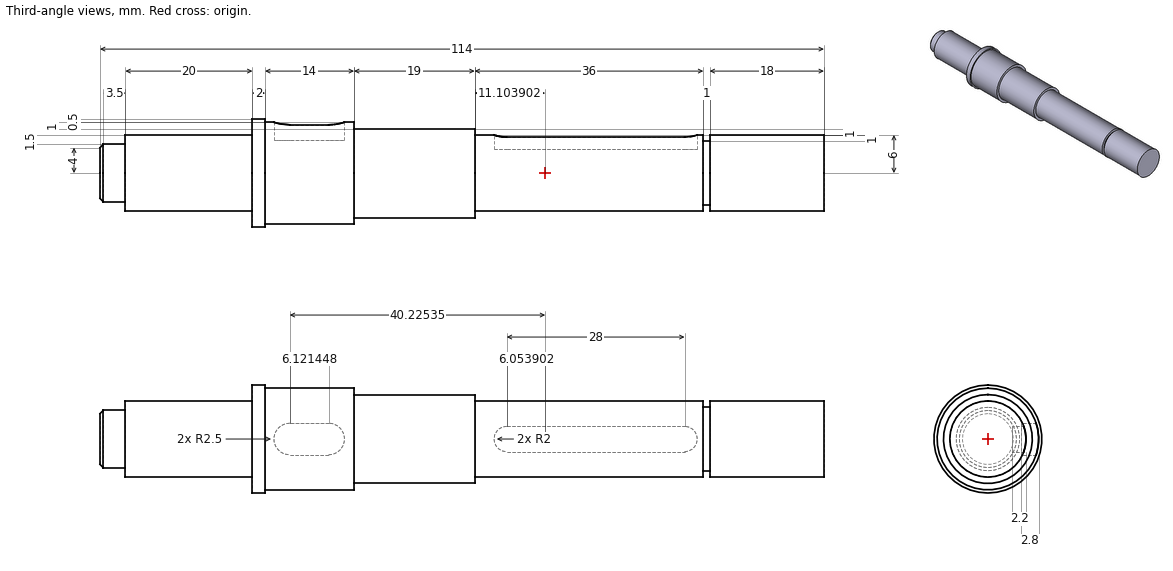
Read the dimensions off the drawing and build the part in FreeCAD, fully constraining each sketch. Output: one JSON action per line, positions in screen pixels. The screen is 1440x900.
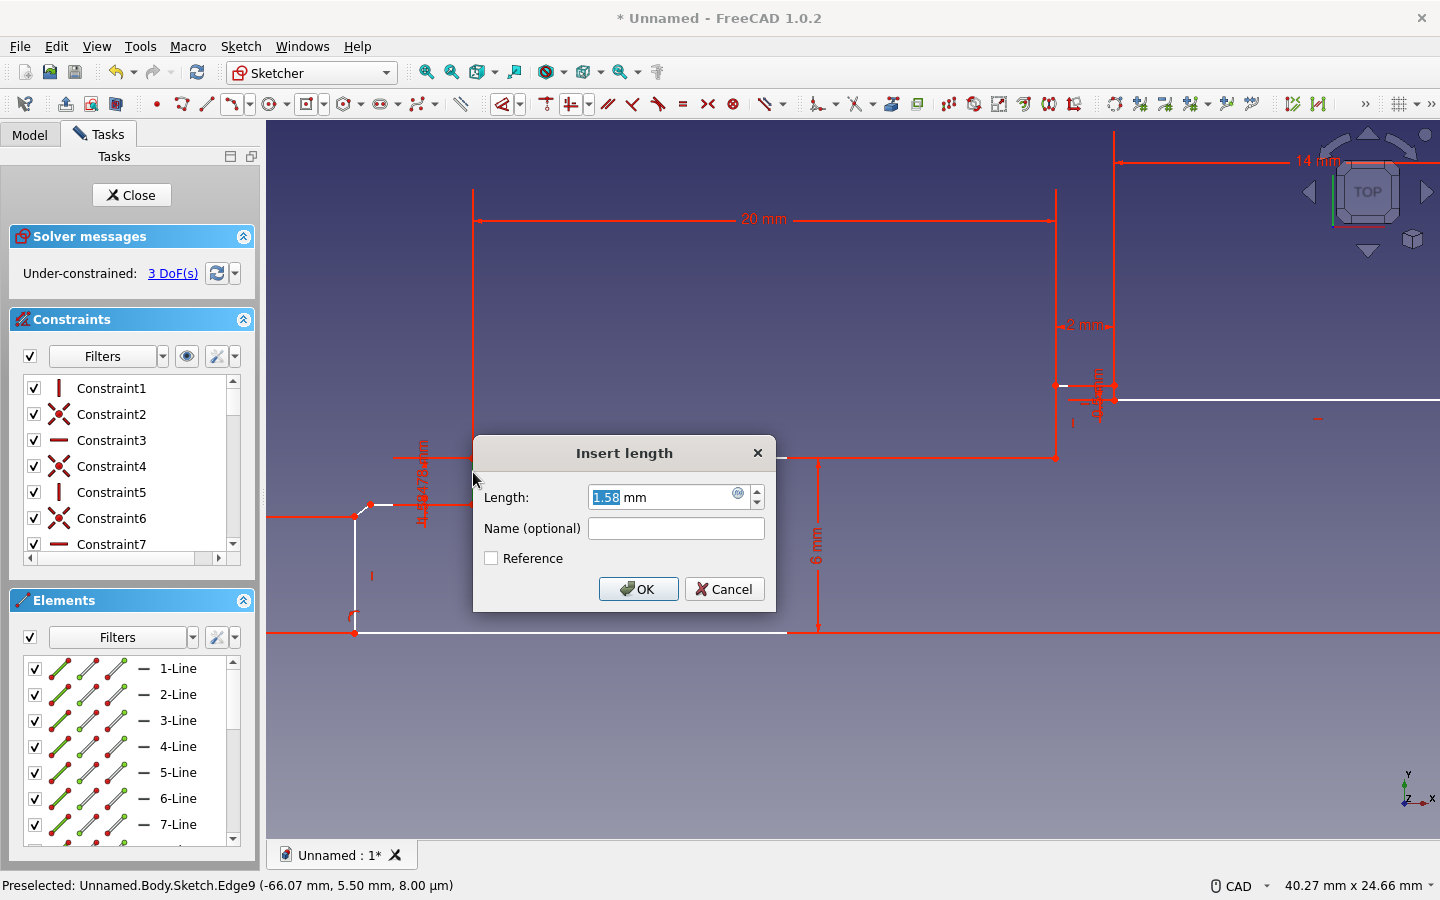
{"action": "type", "text": "1.5"}
{"action": "key", "text": "Return"}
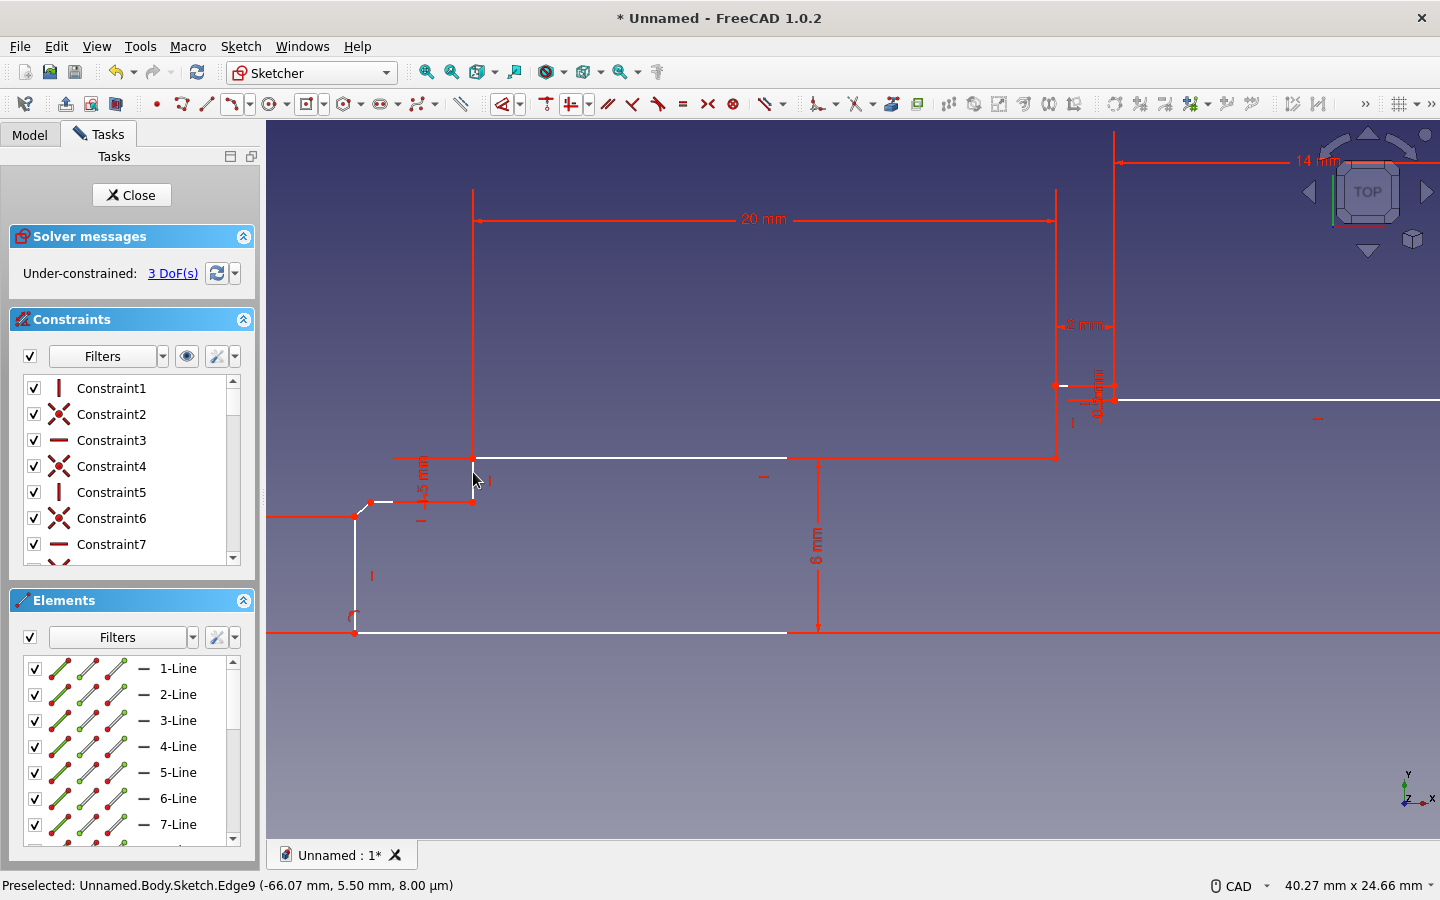
{"action": "left_click", "coordinate": [442, 502]}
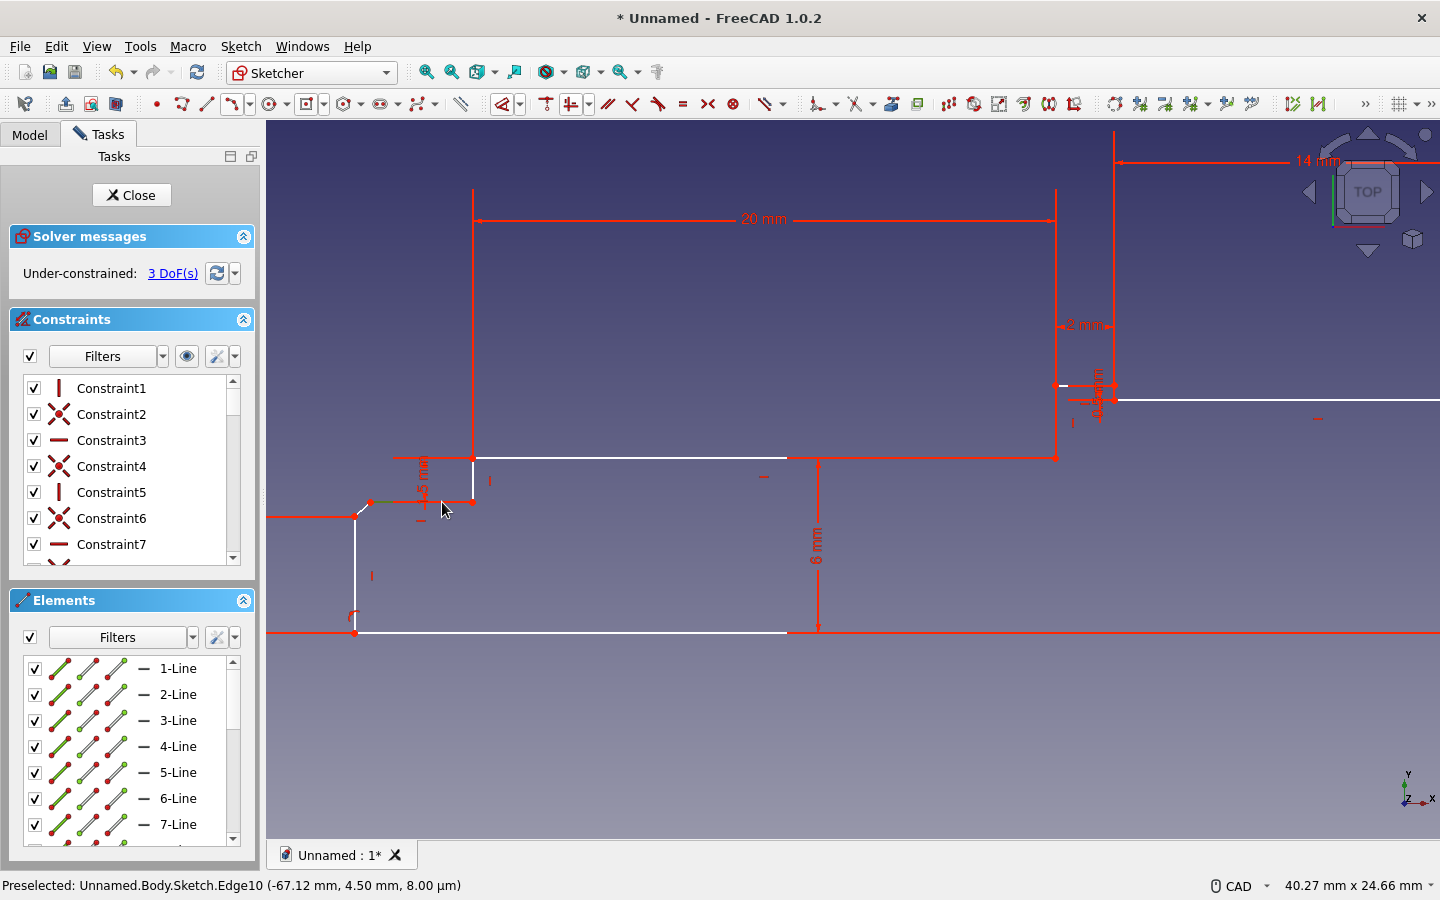
{"action": "key", "text": "l"}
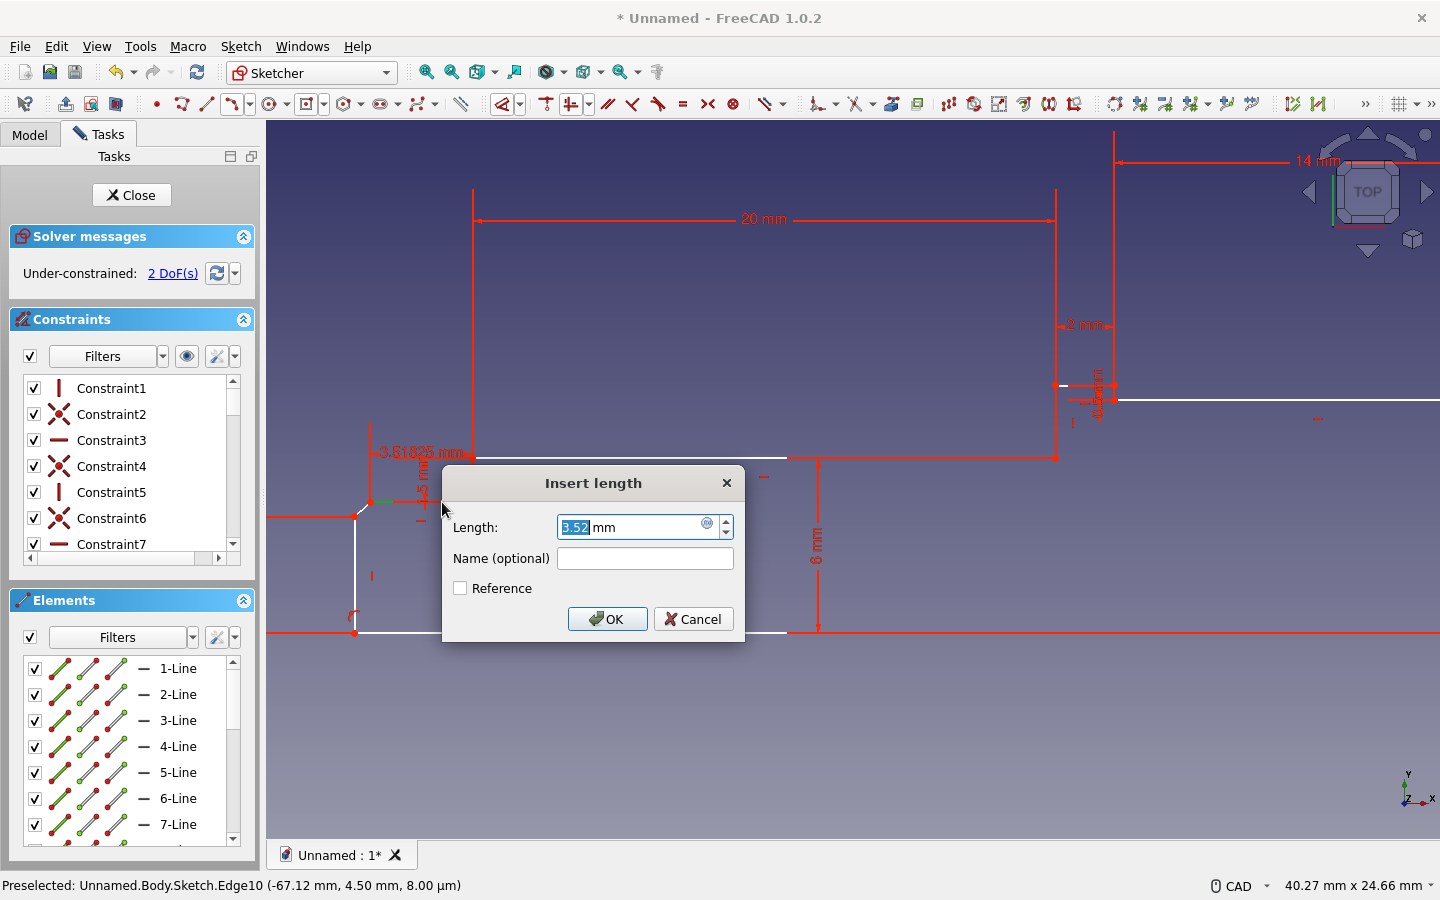
{"action": "type", "text": "3.5"}
{"action": "key", "text": "Return"}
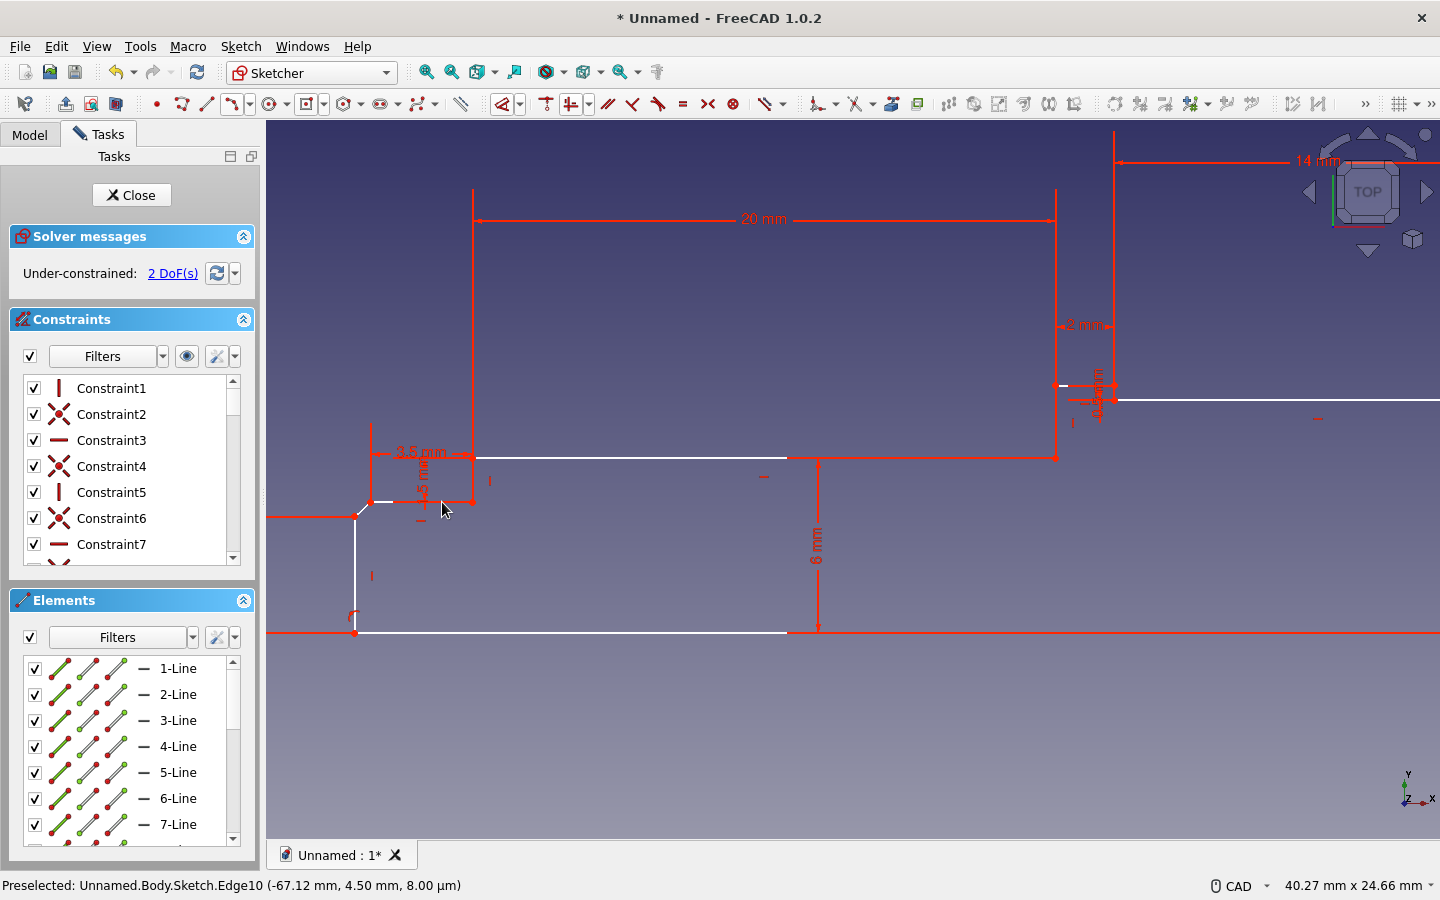
{"action": "scroll", "coordinate": [473, 472], "scroll_direction": "down", "scroll_amount": 8}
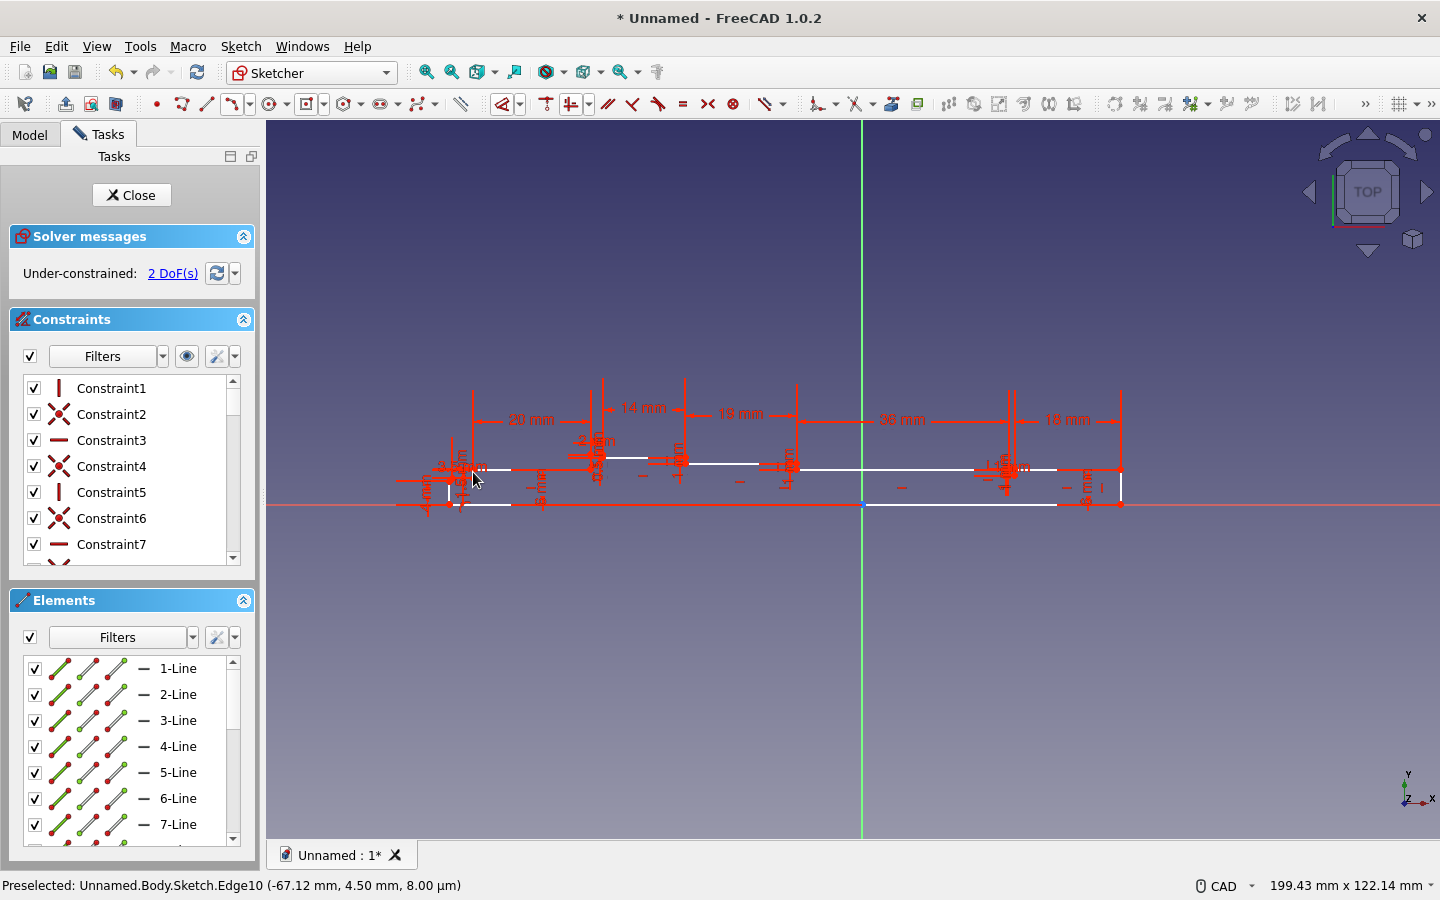
{"action": "left_click", "coordinate": [584, 505]}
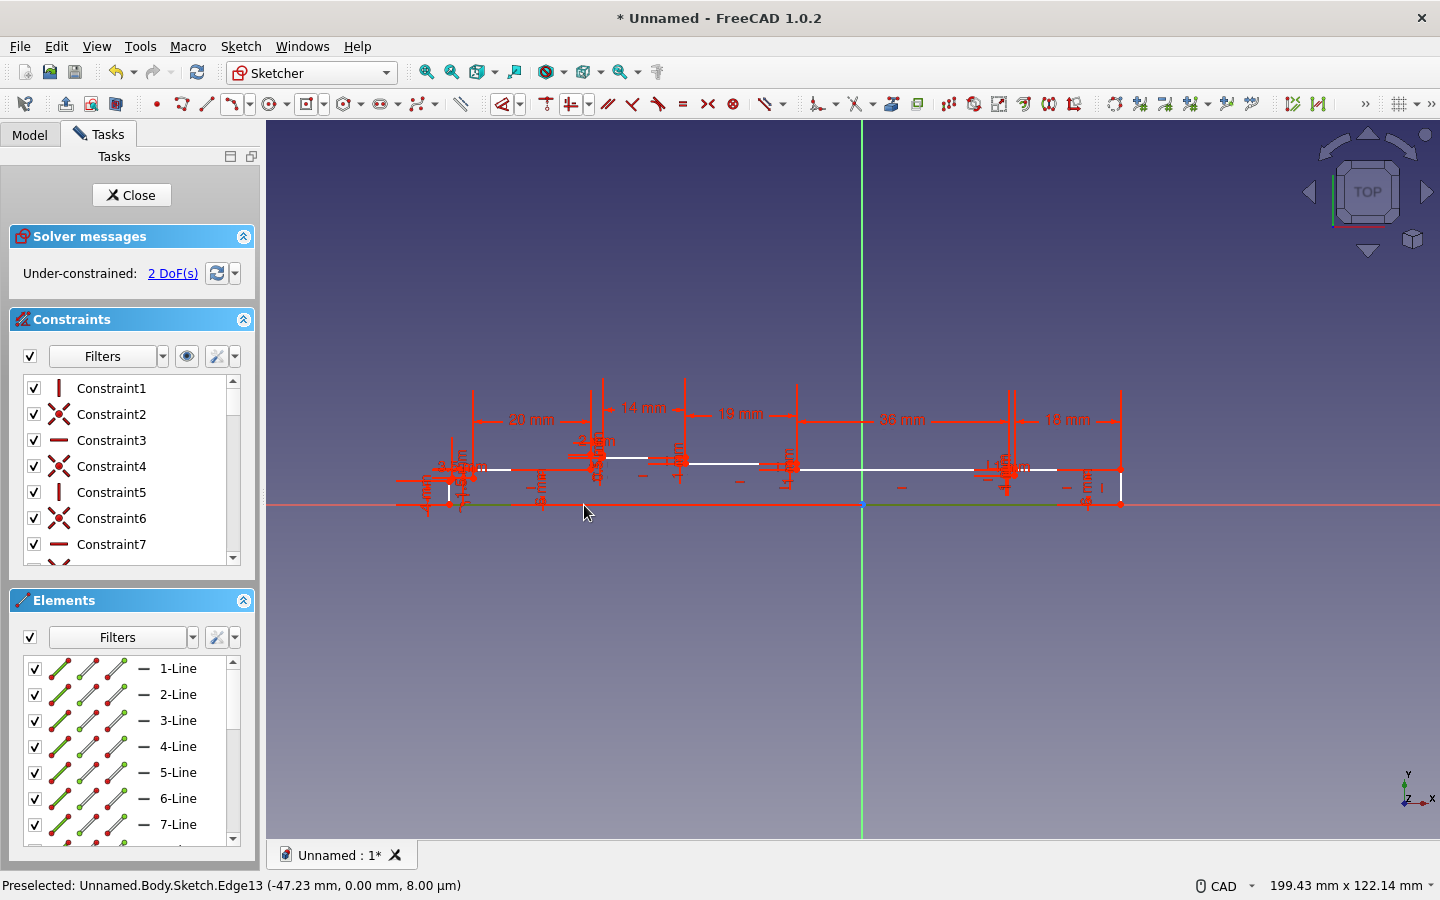
{"action": "key", "text": "l"}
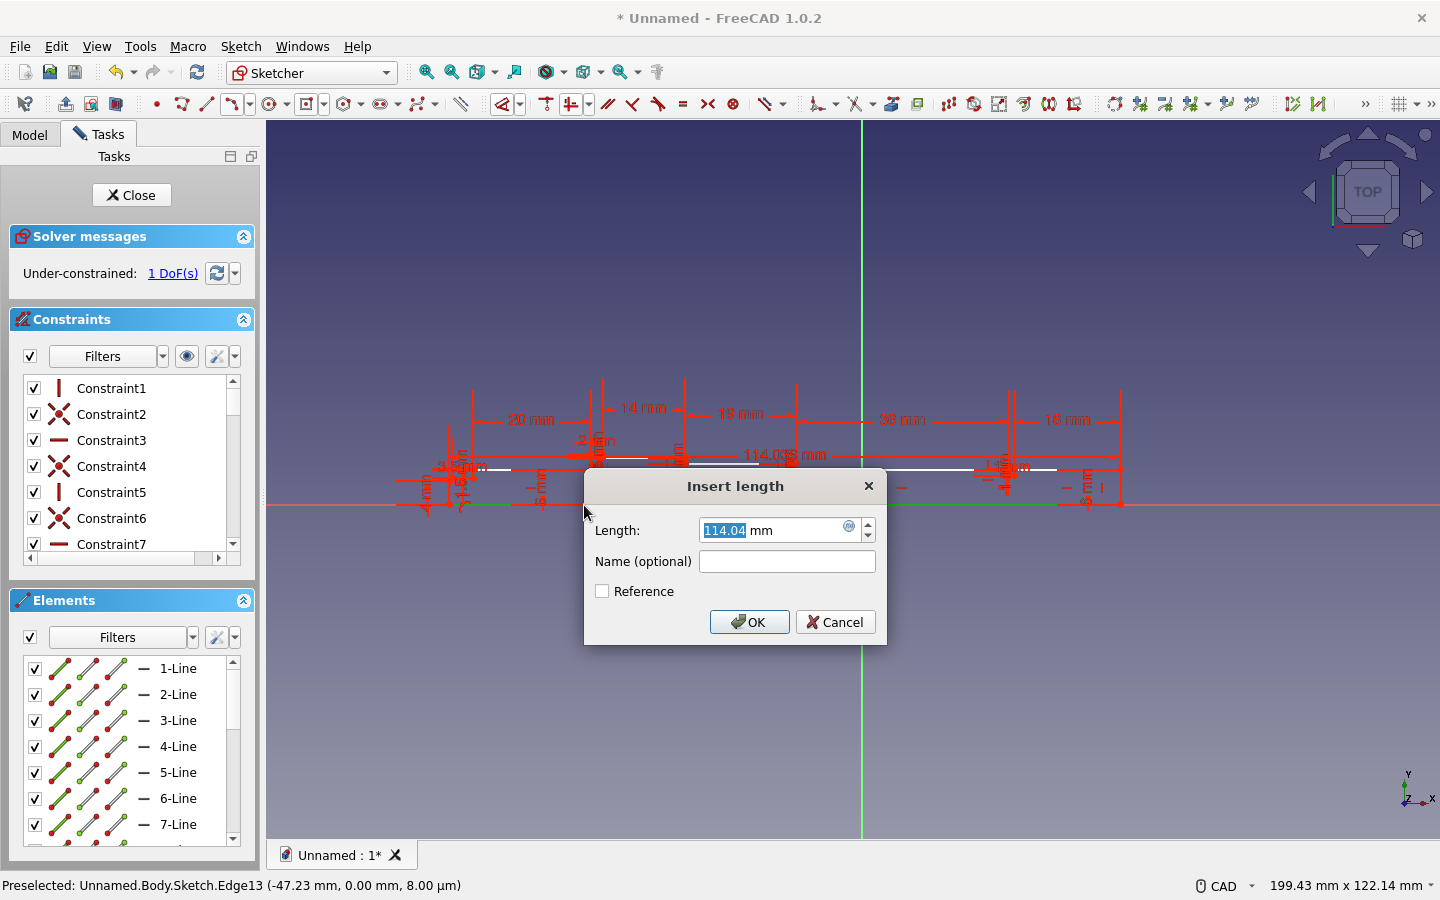
{"action": "type", "text": "114"}
{"action": "key", "text": "Return"}